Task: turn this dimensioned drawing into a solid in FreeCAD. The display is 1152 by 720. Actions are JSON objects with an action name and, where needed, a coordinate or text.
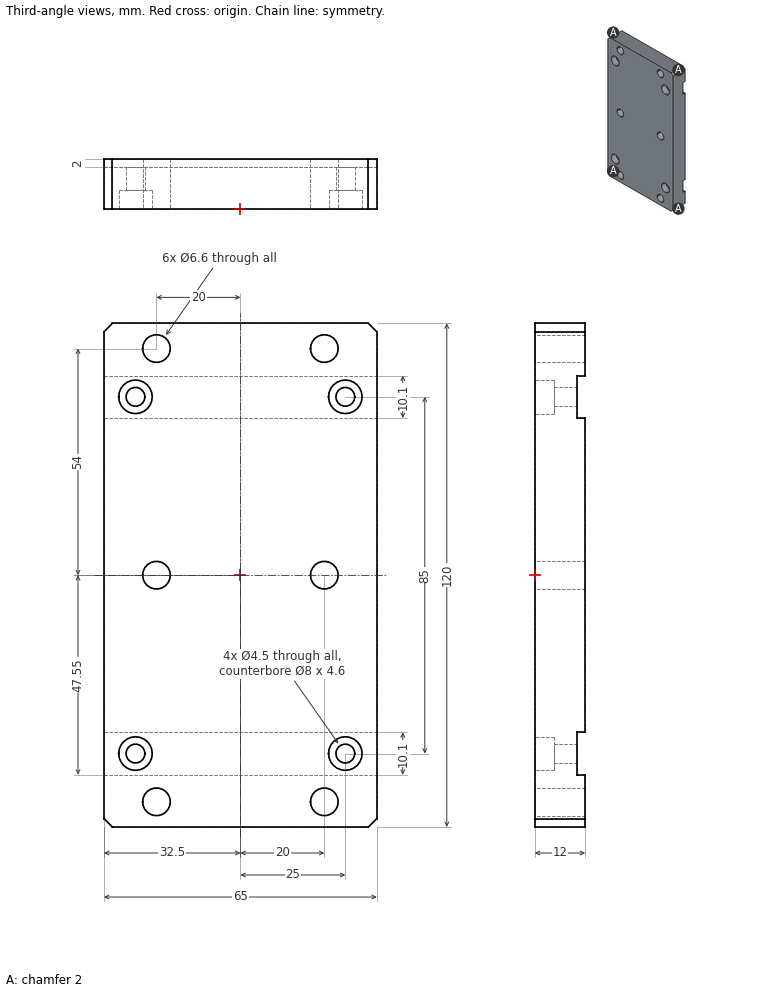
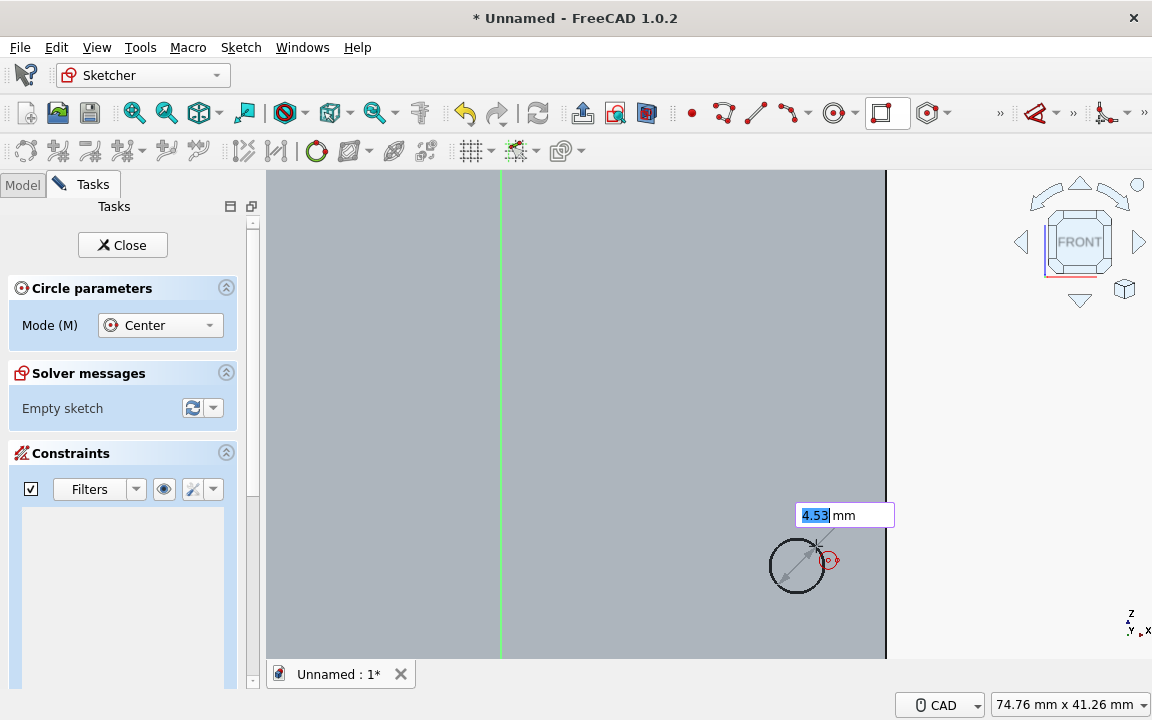
{"action": "type", "text": "4.5"}
{"action": "key", "text": "Return"}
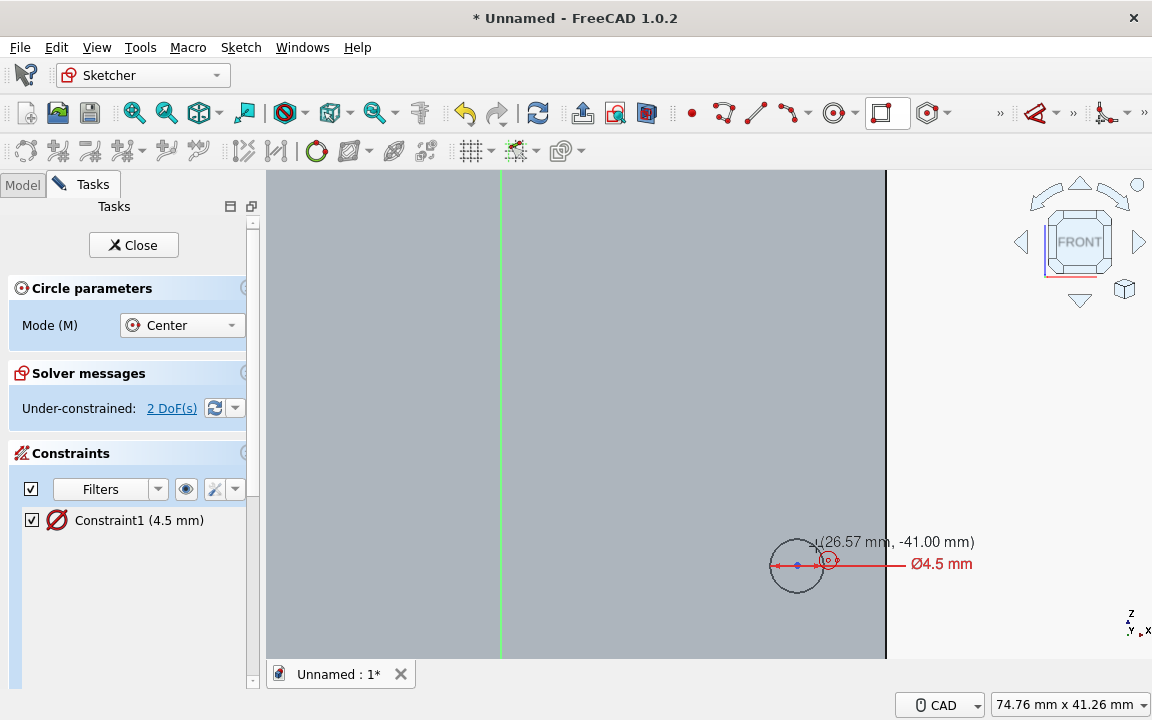
{"action": "scroll", "coordinate": [701, 567], "scroll_direction": "down", "scroll_amount": 6}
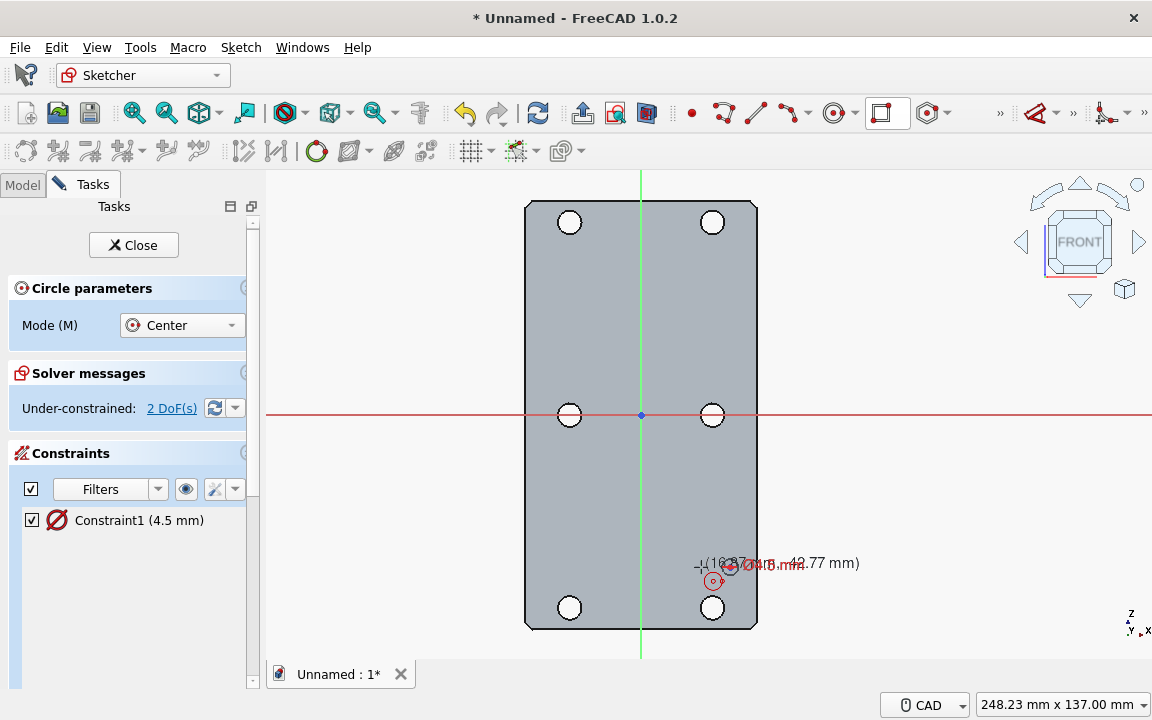
{"action": "scroll", "coordinate": [730, 264], "scroll_direction": "up", "scroll_amount": 6}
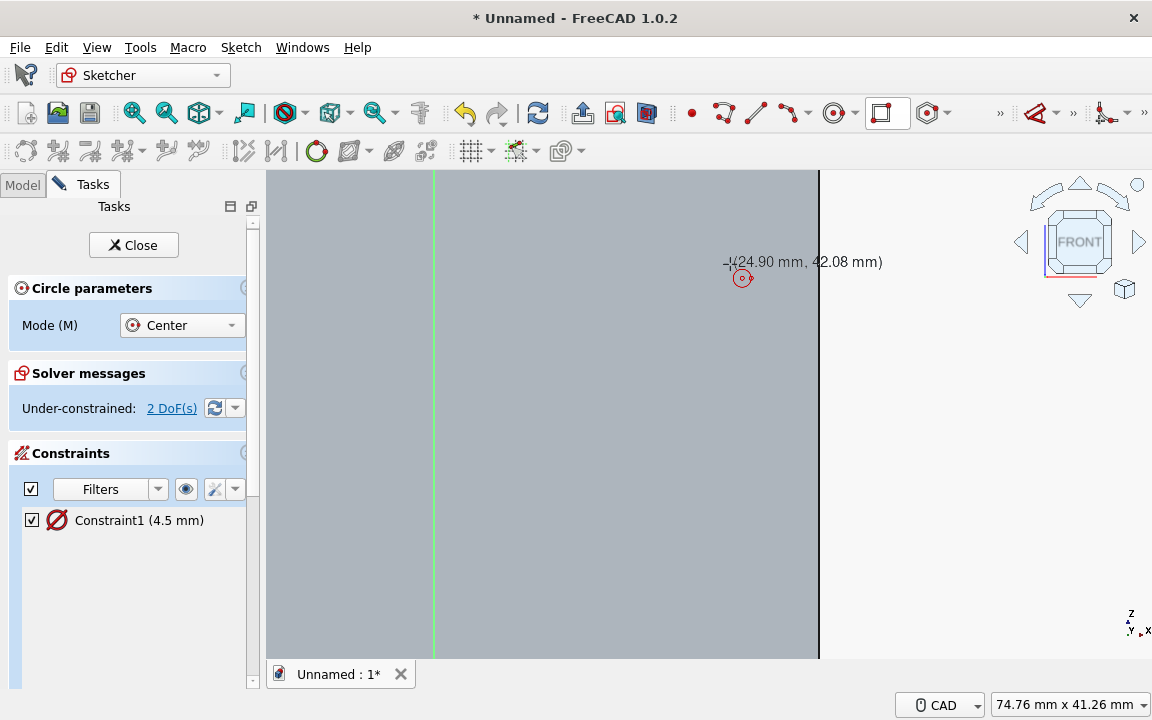
{"action": "left_click", "coordinate": [730, 262]}
{"action": "mouse_move", "coordinate": [749, 243]}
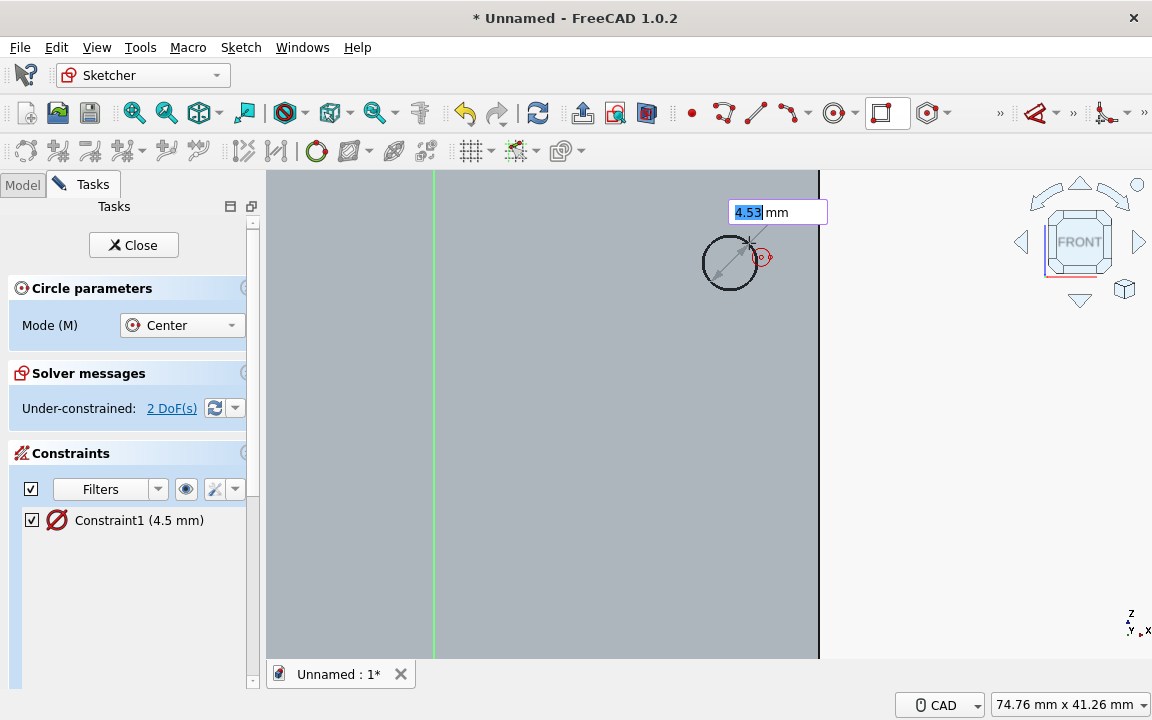
{"action": "type", "text": "4.5"}
{"action": "key", "text": "Return"}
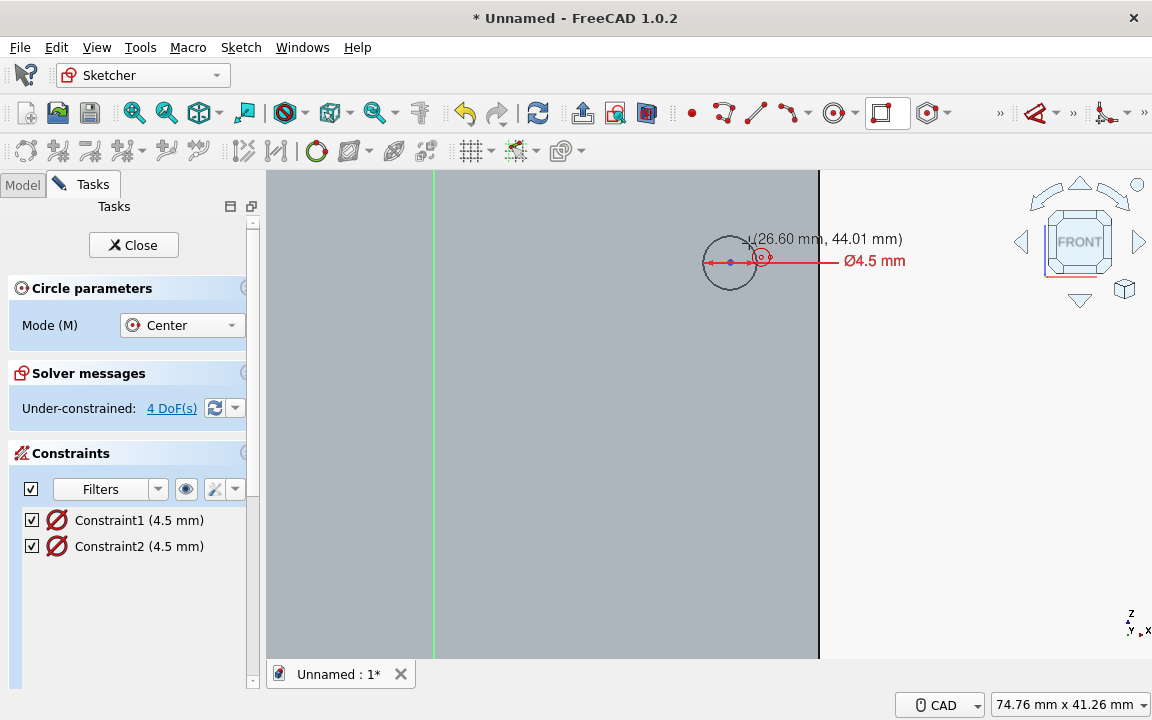
{"action": "scroll", "coordinate": [730, 263], "scroll_direction": "down", "scroll_amount": 6}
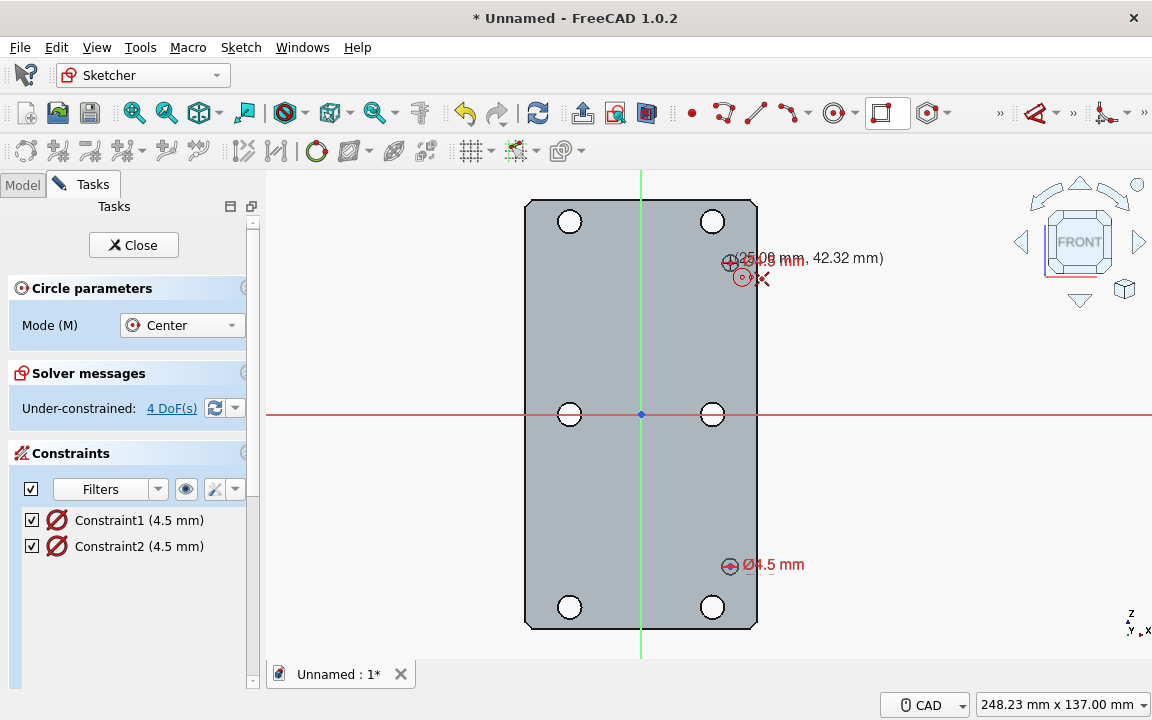
{"action": "scroll", "coordinate": [552, 263], "scroll_direction": "up", "scroll_amount": 6}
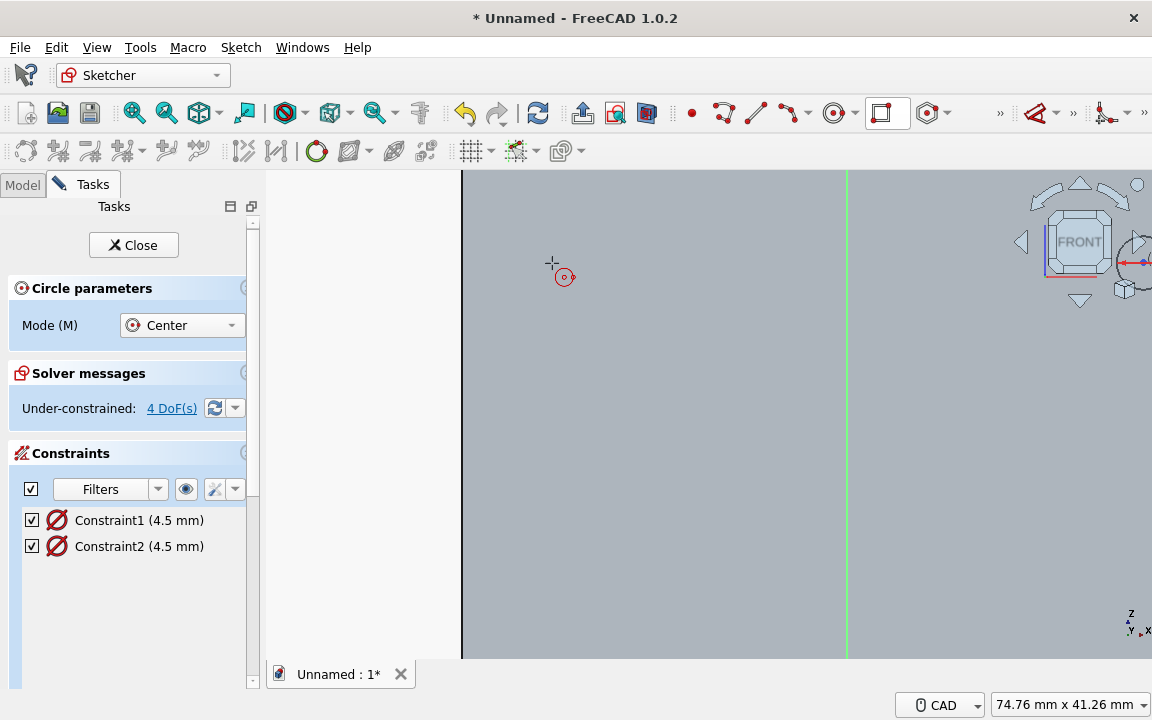
{"action": "left_click", "coordinate": [551, 262]}
{"action": "mouse_move", "coordinate": [570, 243]}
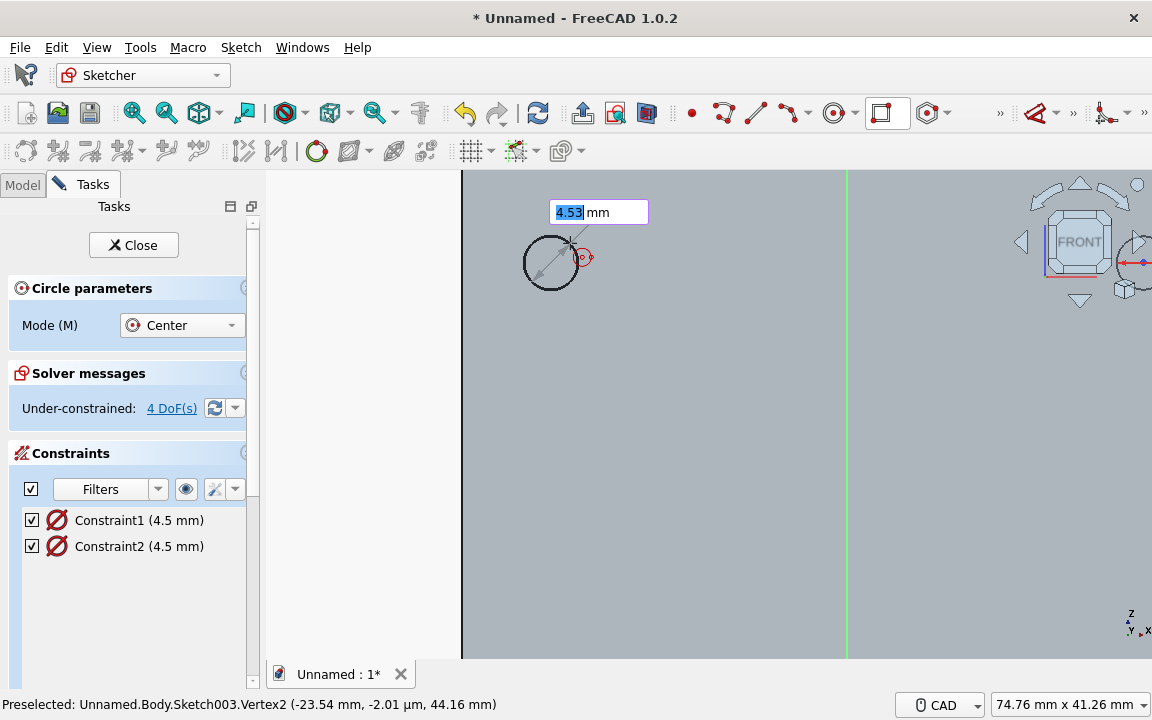
{"action": "type", "text": "4.5"}
{"action": "key", "text": "Return"}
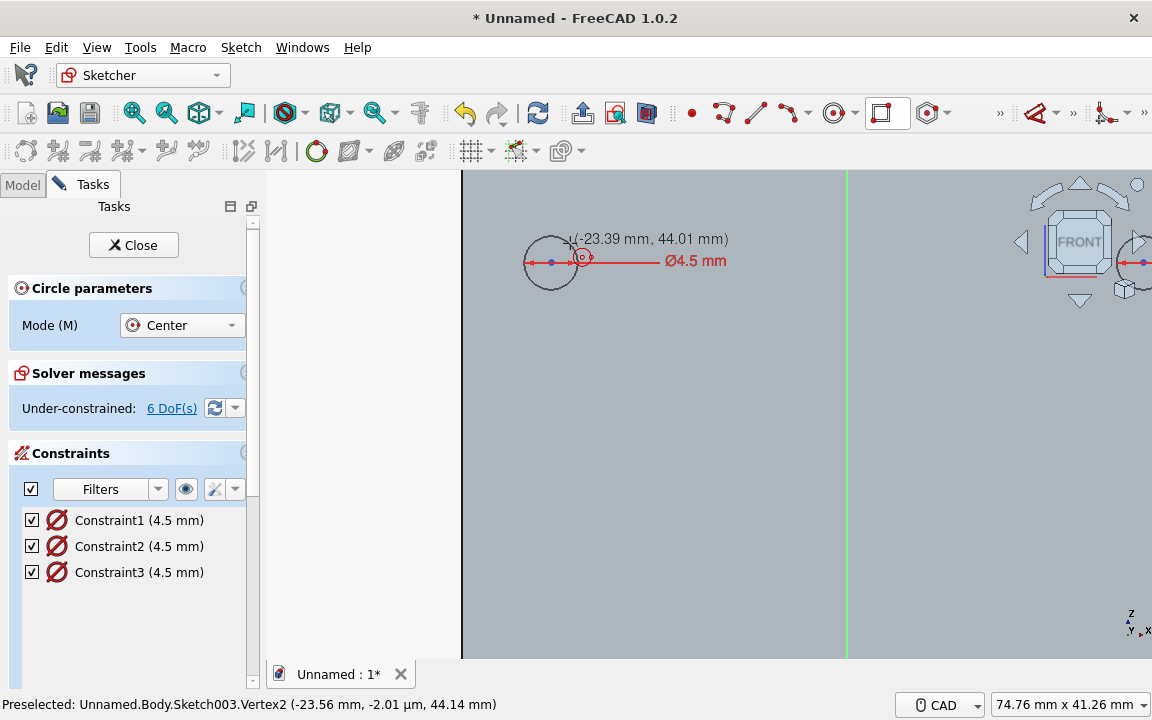
{"action": "scroll", "coordinate": [551, 263], "scroll_direction": "down", "scroll_amount": 6}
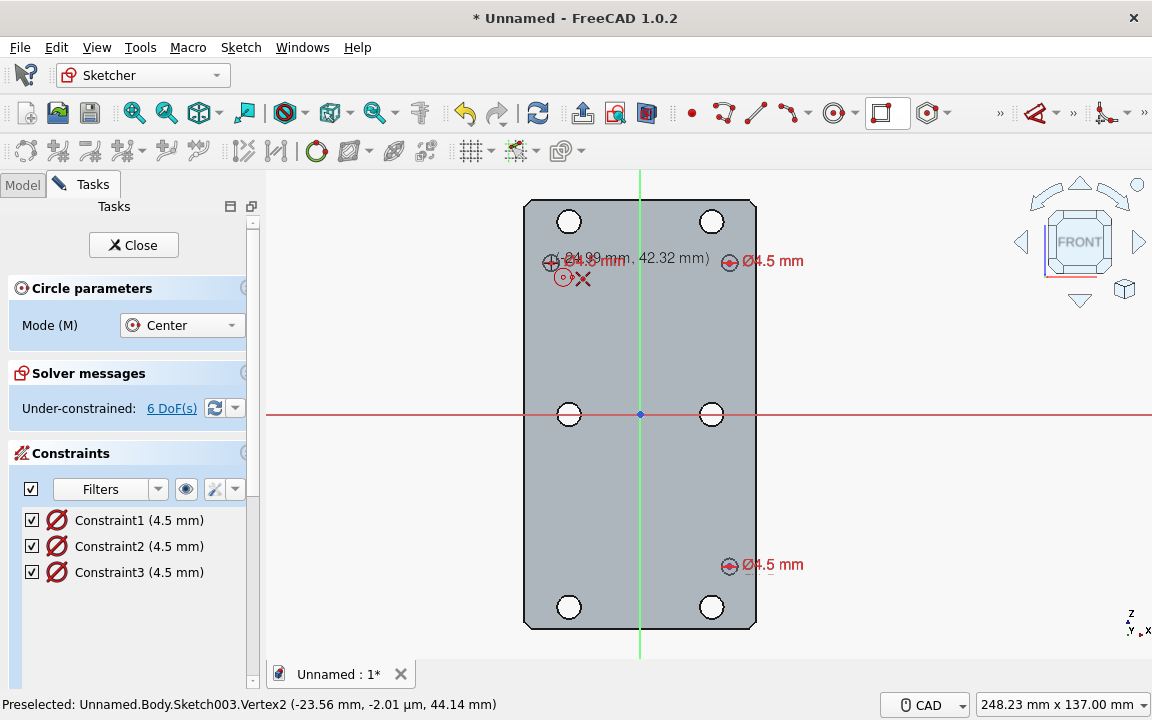
{"action": "scroll", "coordinate": [551, 566], "scroll_direction": "up", "scroll_amount": 6}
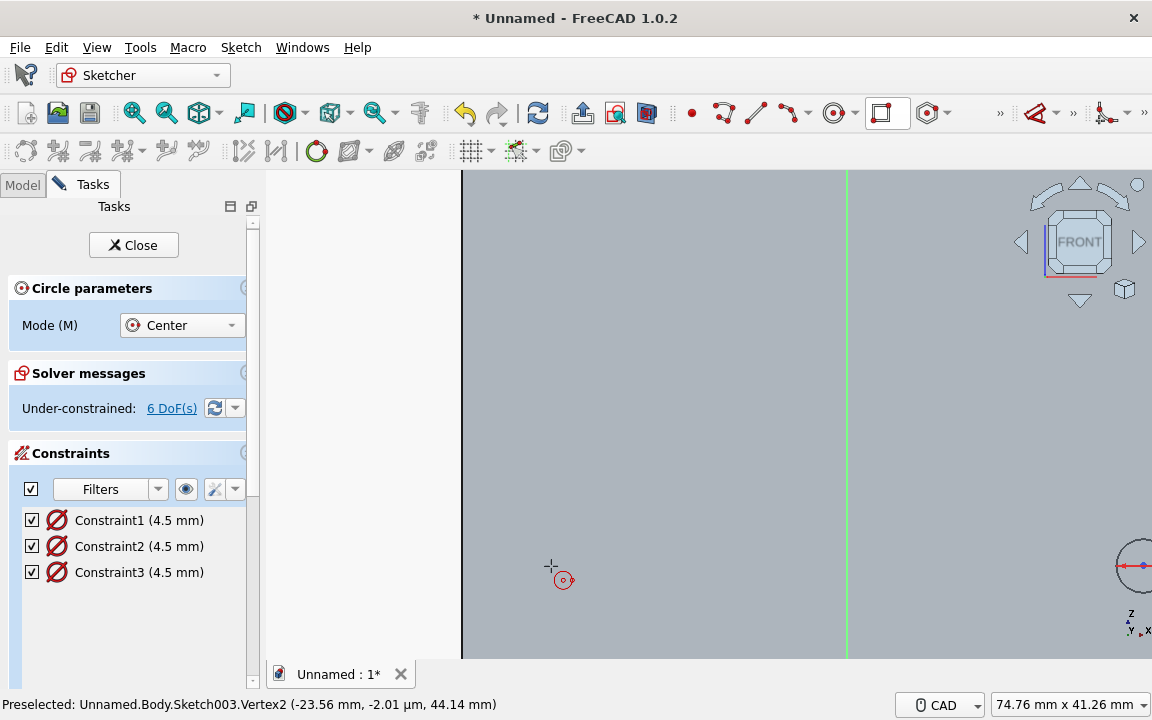
{"action": "left_click", "coordinate": [551, 565]}
{"action": "mouse_move", "coordinate": [570, 546]}